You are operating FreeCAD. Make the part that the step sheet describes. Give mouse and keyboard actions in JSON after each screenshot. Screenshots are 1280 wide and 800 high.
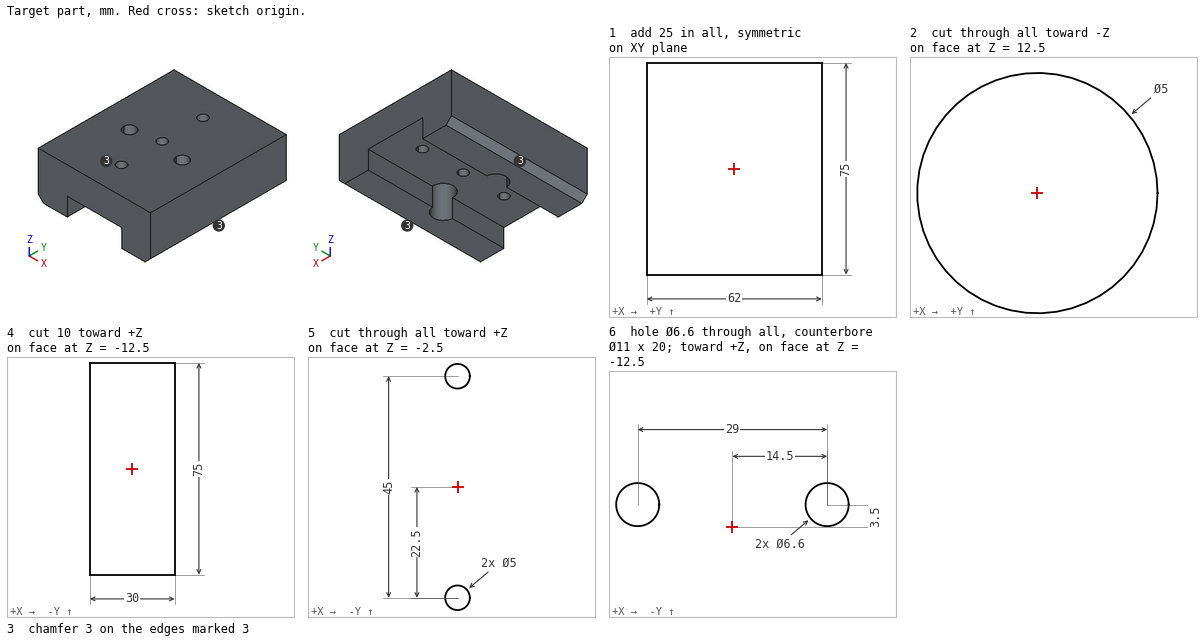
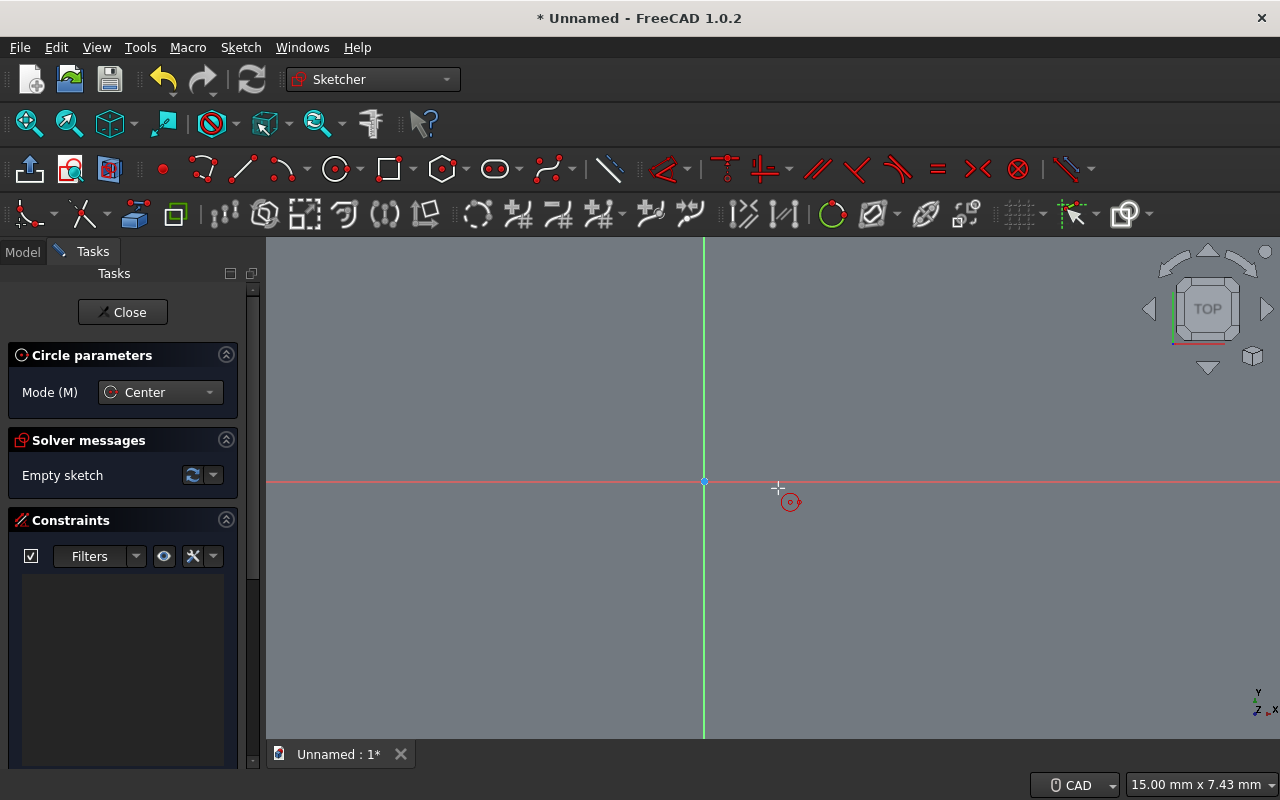
{"action": "left_click", "coordinate": [704, 482]}
{"action": "left_click", "coordinate": [824, 362]}
{"action": "key", "text": "Escape"}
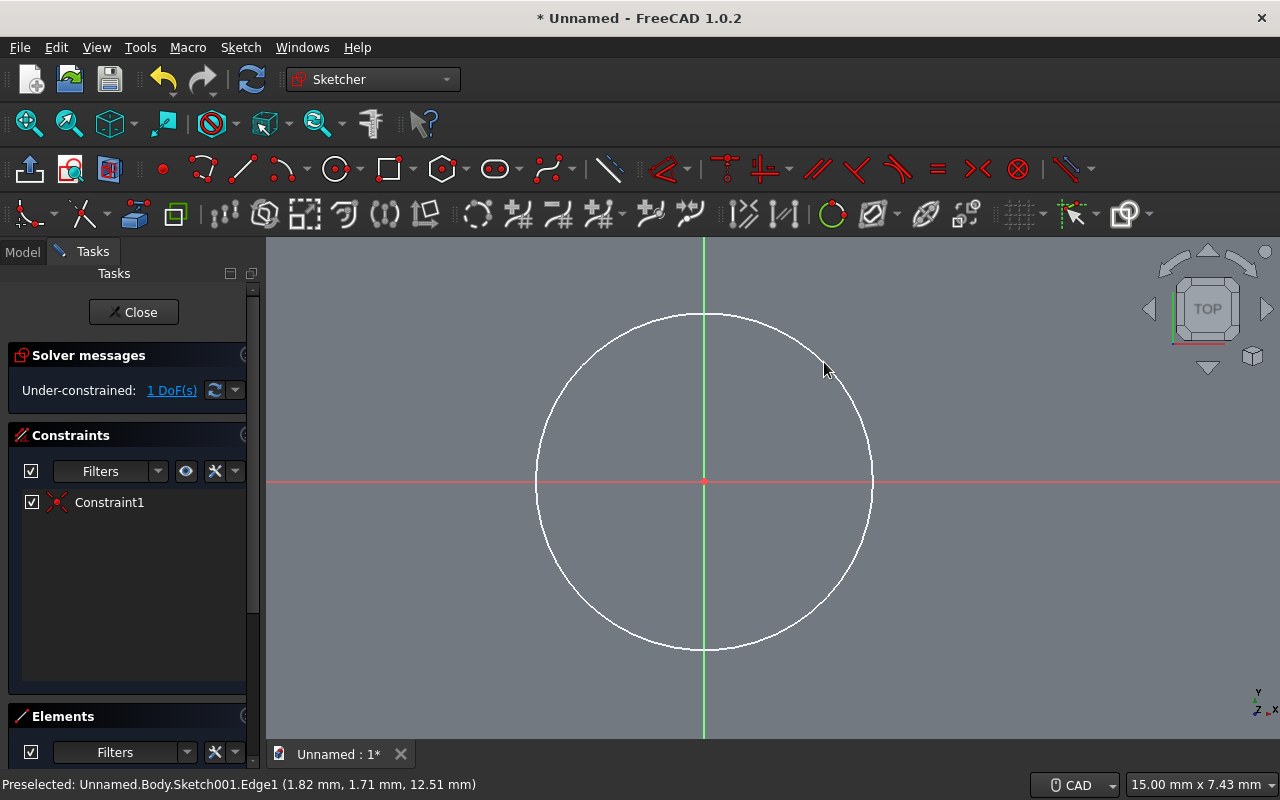
{"action": "left_click", "coordinate": [664, 170]}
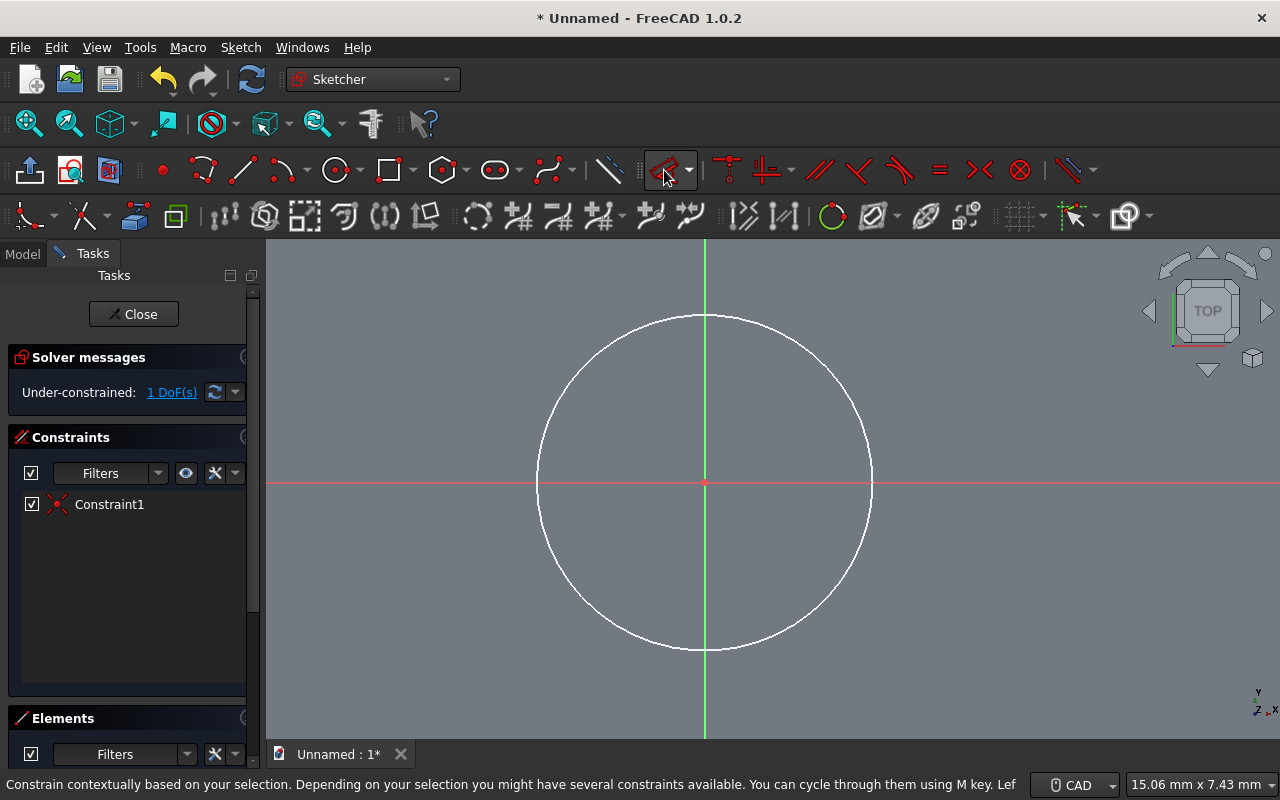
{"action": "left_click", "coordinate": [823, 364]}
{"action": "left_click", "coordinate": [846, 341]}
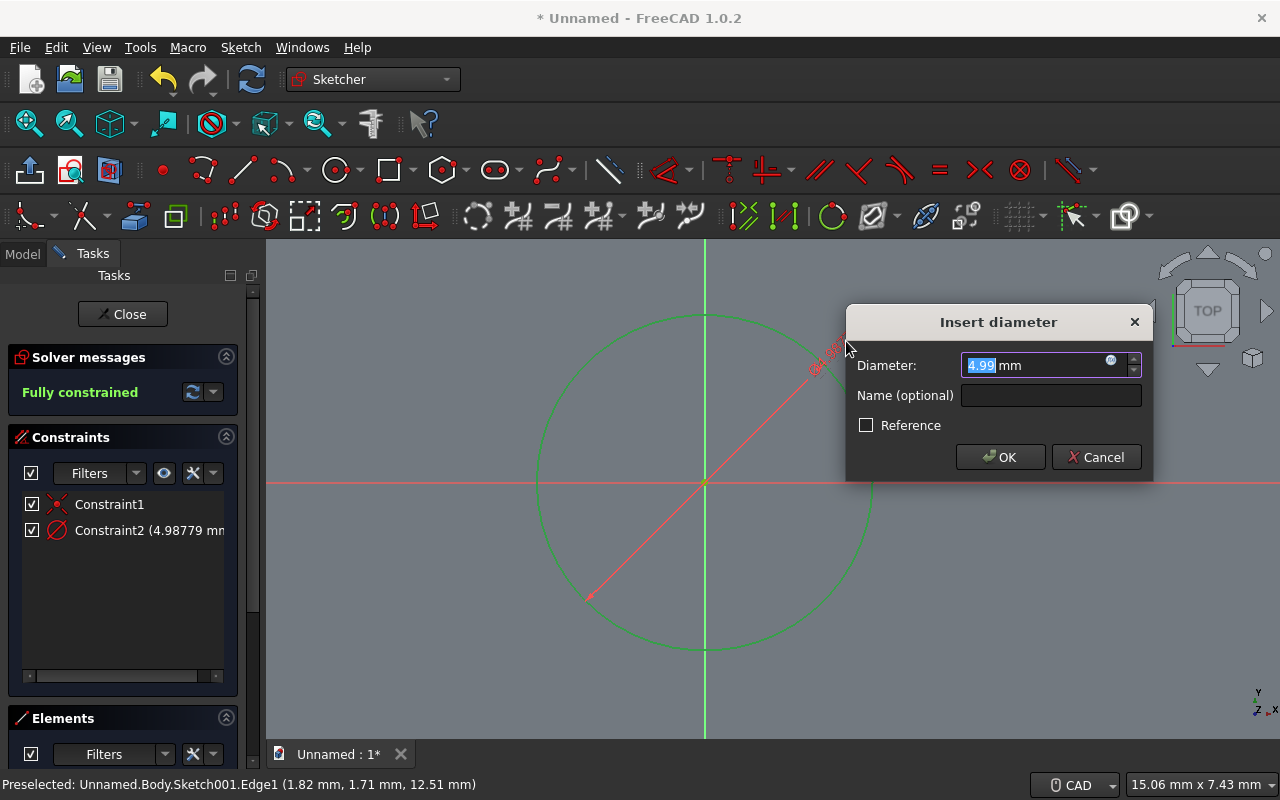
{"action": "type", "text": "5"}
{"action": "key", "text": "Return"}
{"action": "key", "text": "Escape"}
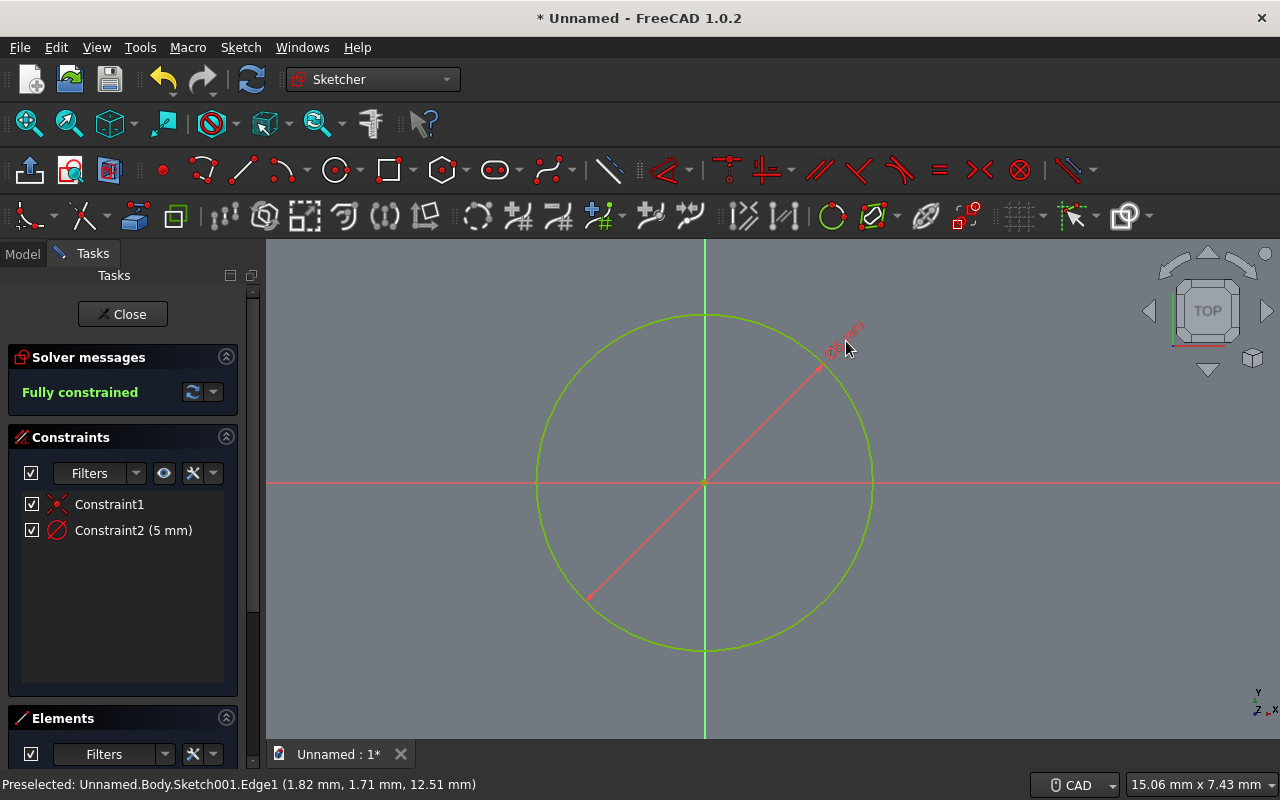
{"action": "left_click", "coordinate": [123, 314]}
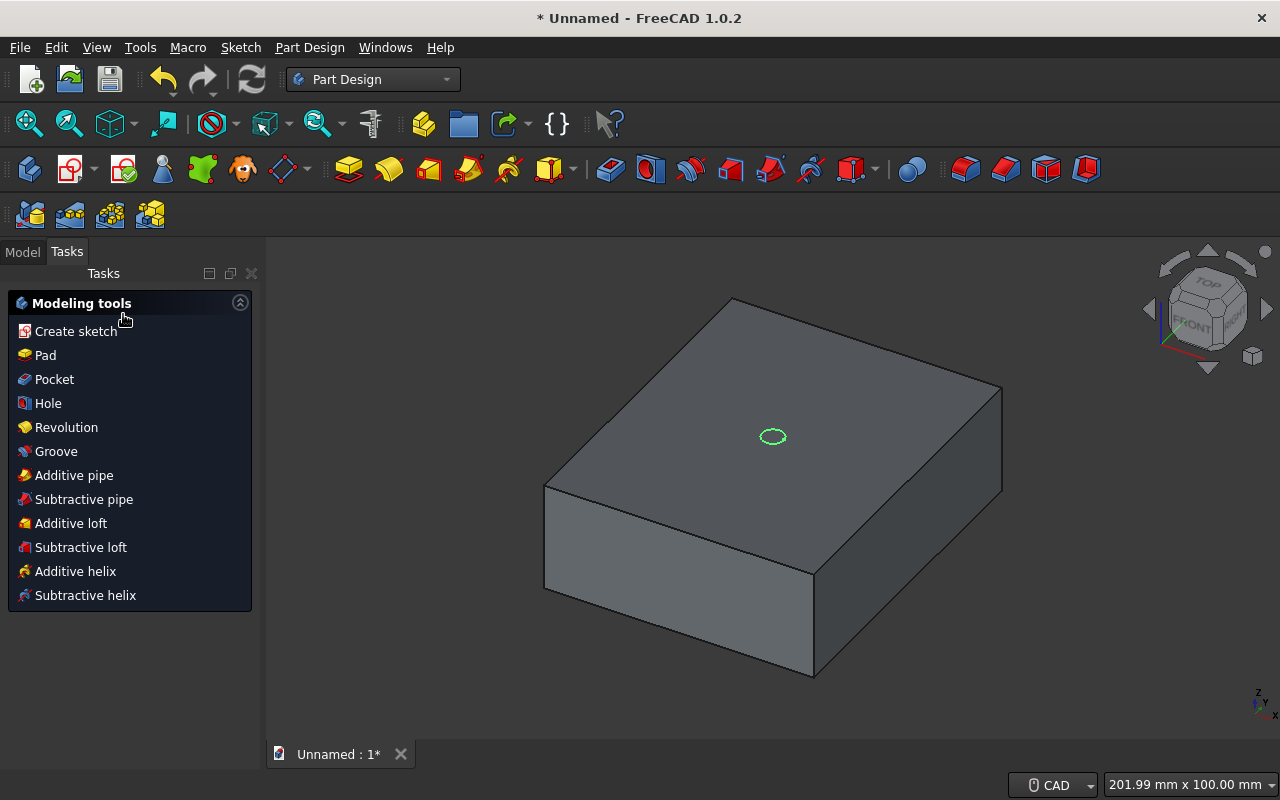
{"action": "left_click", "coordinate": [612, 170]}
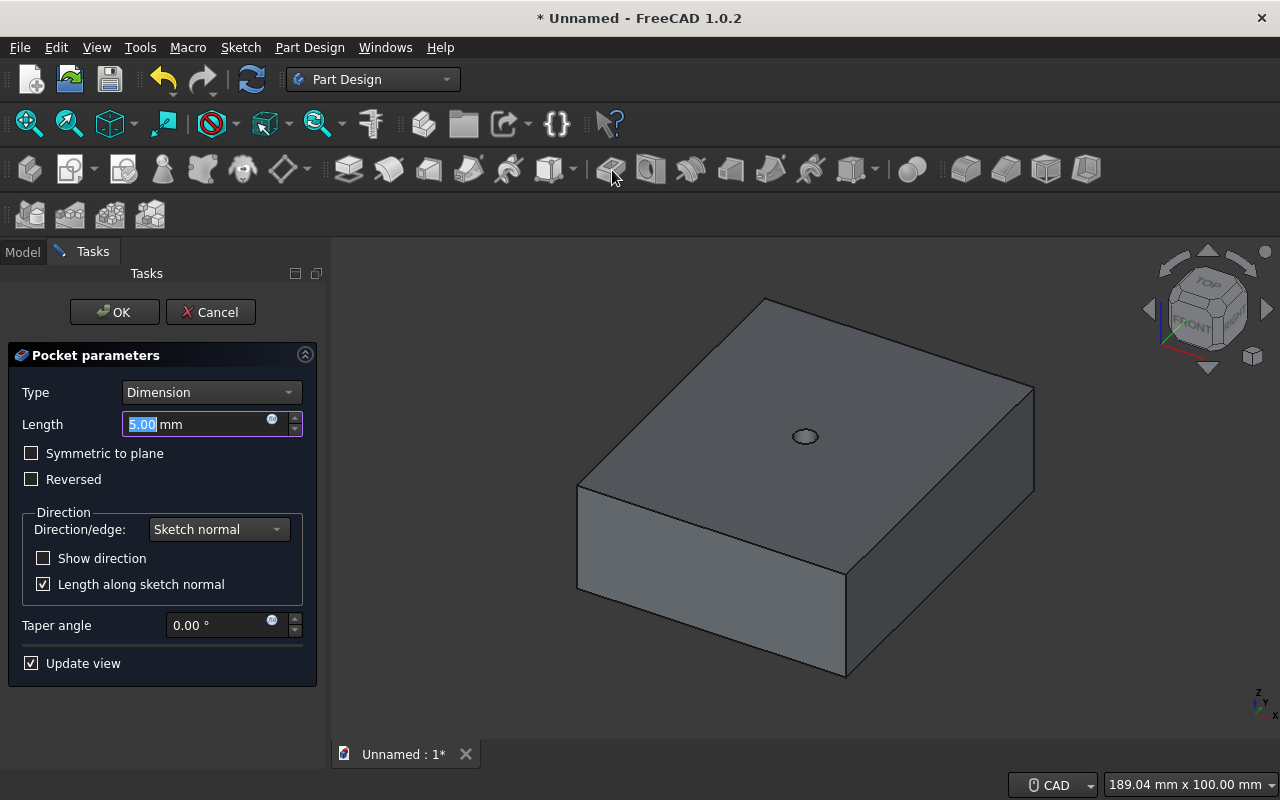
{"action": "left_click", "coordinate": [212, 392]}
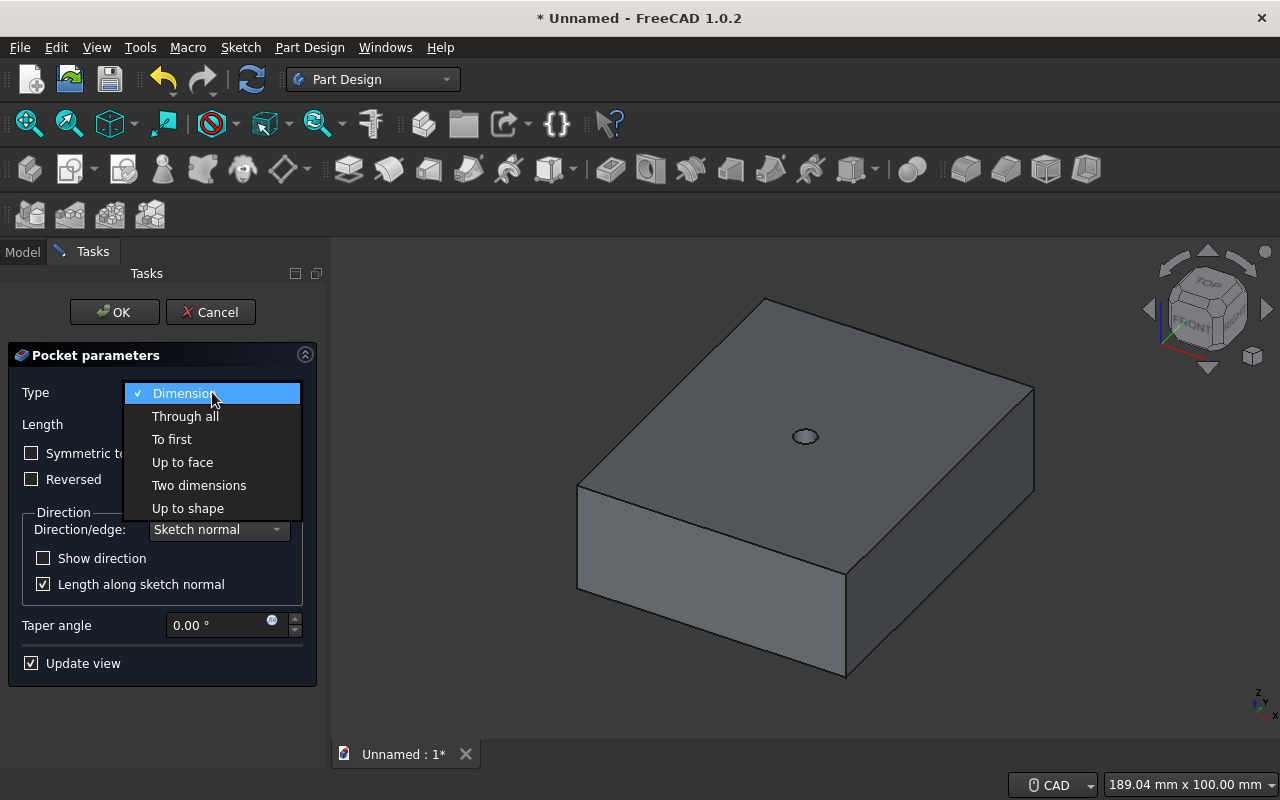
{"action": "left_click", "coordinate": [212, 416]}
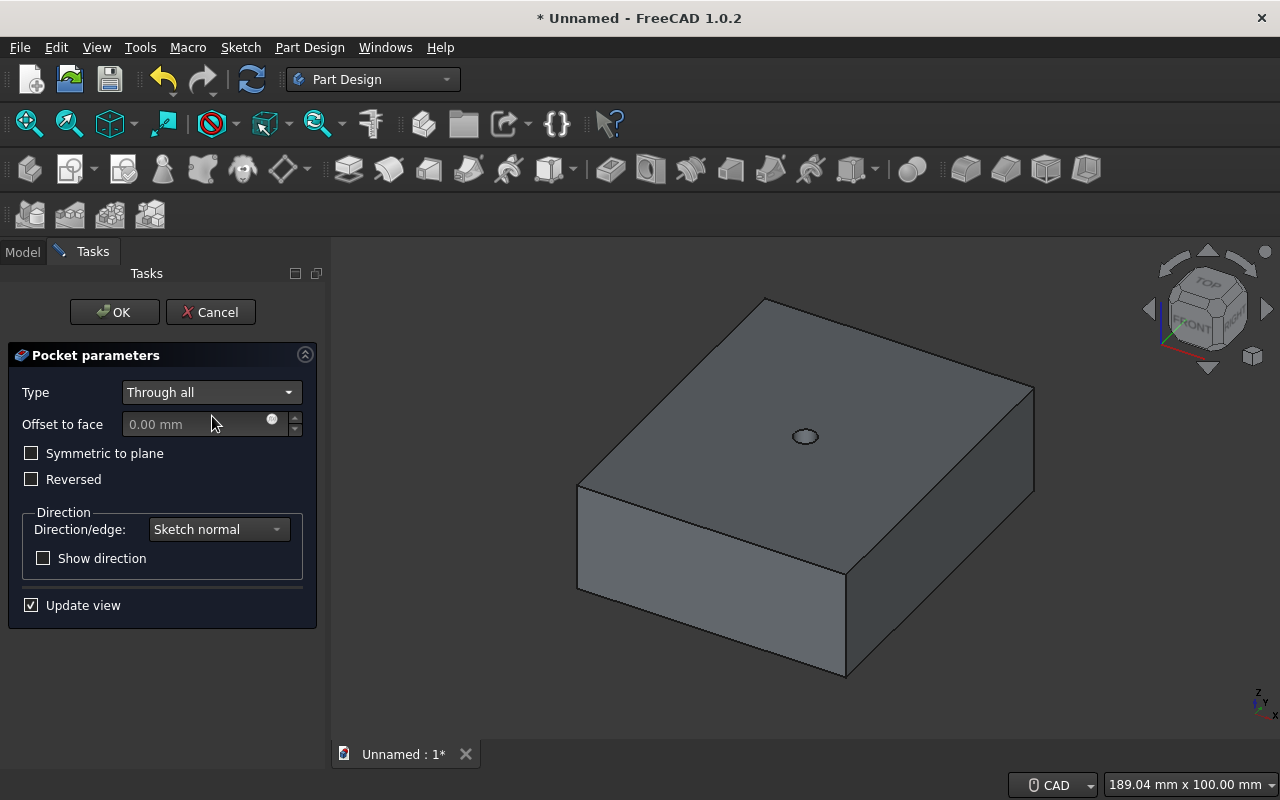
{"action": "left_click", "coordinate": [115, 312]}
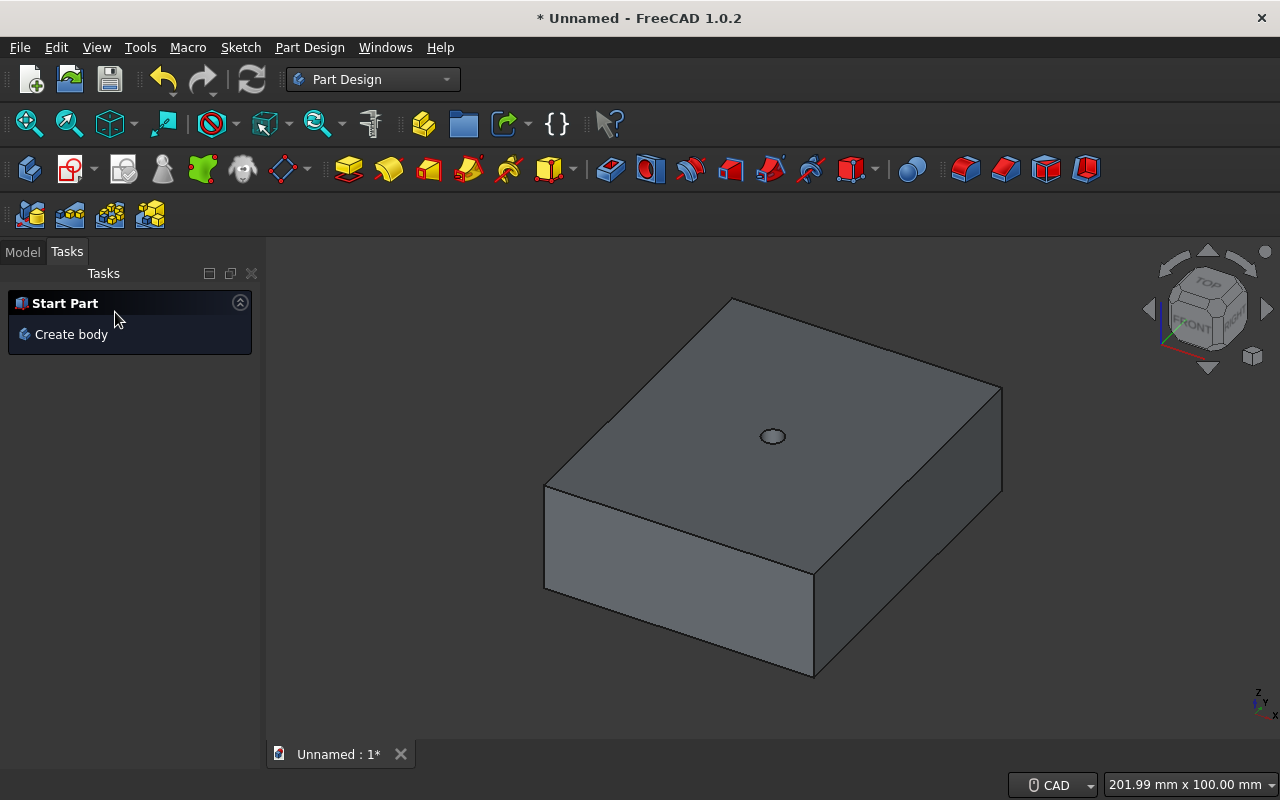
{"action": "key", "text": "0"}